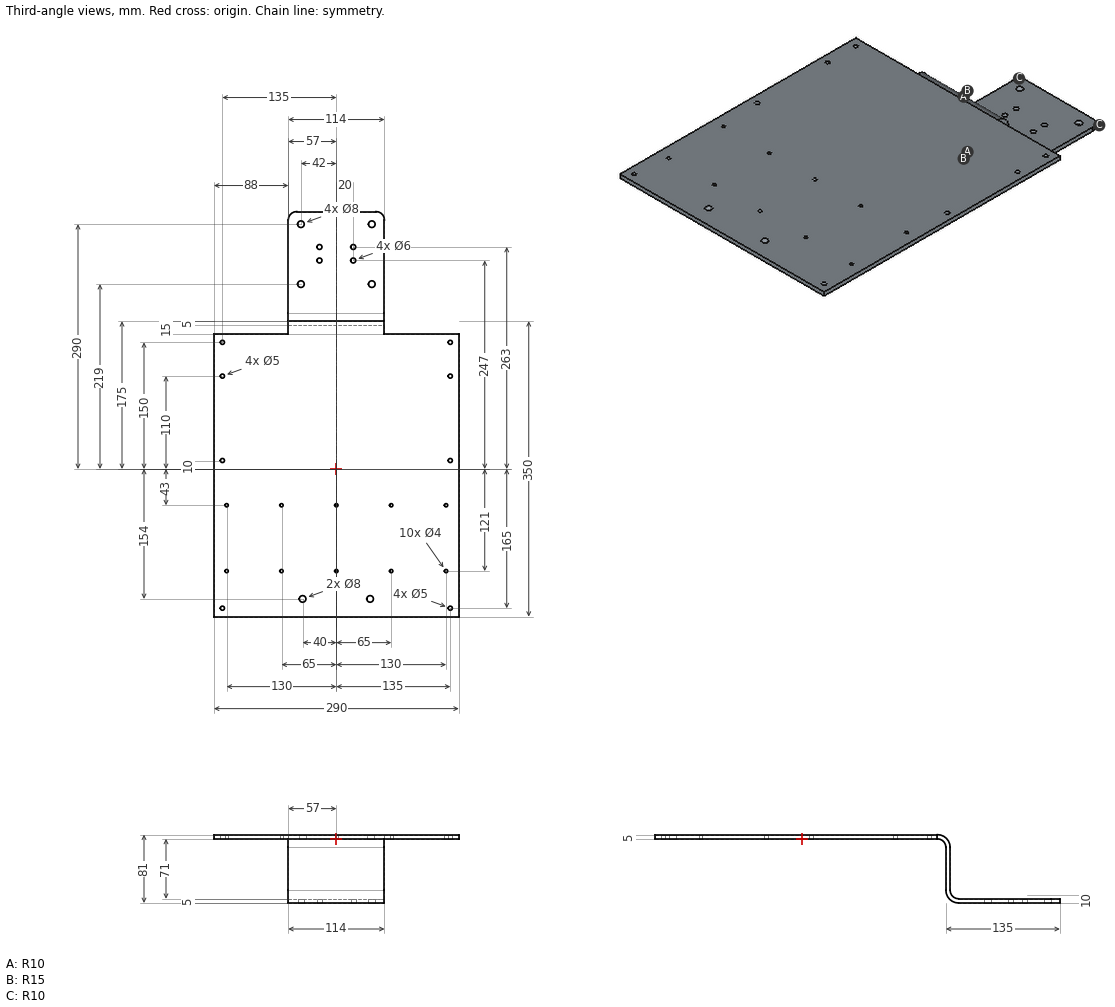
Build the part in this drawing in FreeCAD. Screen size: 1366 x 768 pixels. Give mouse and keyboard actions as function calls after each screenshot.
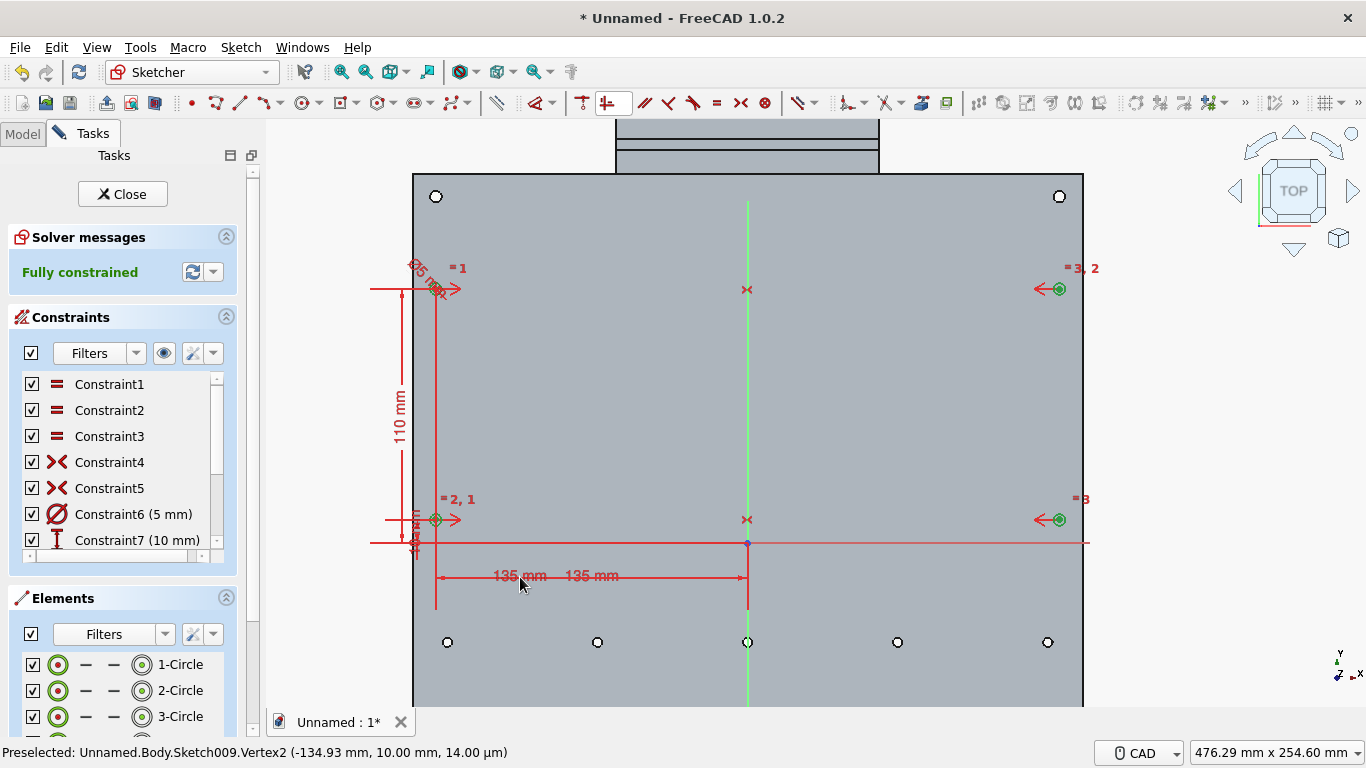
click(123, 194)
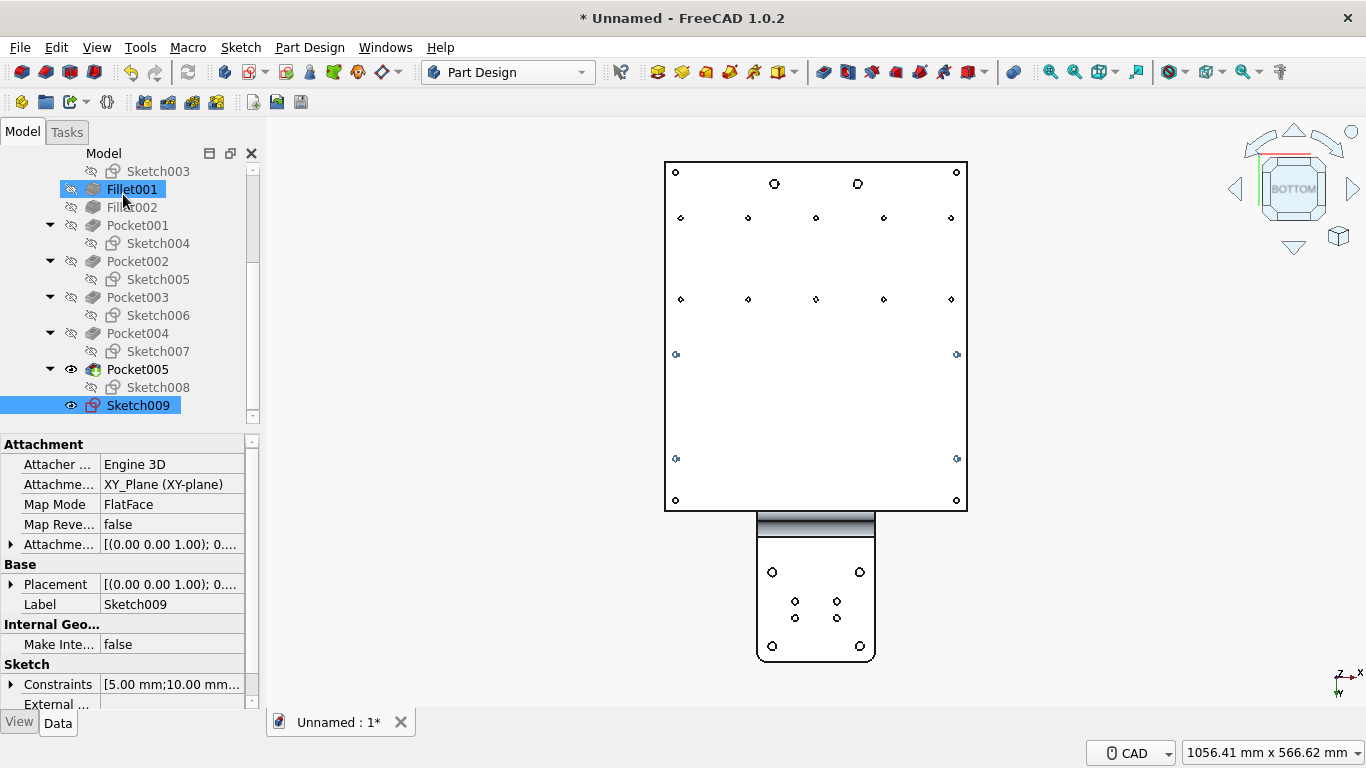
click(824, 72)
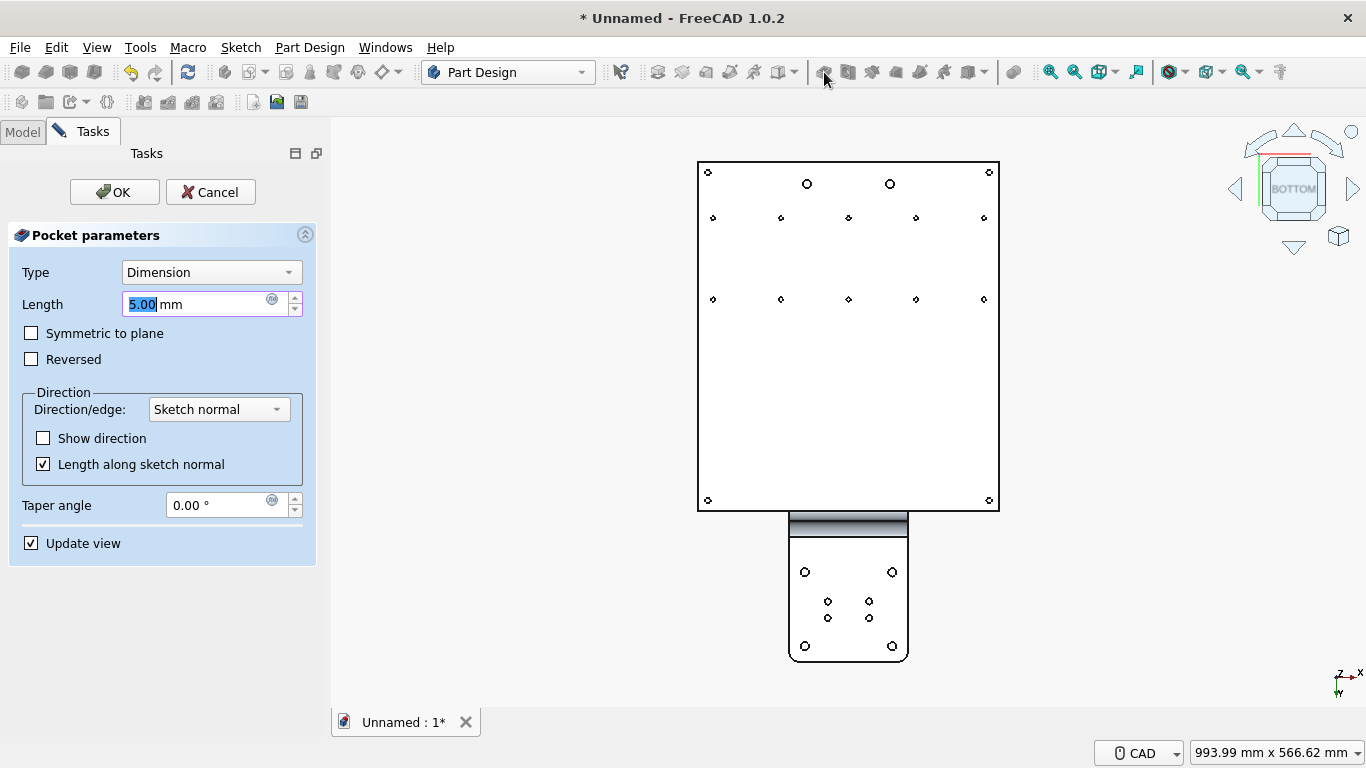
text(10)
key(Tab)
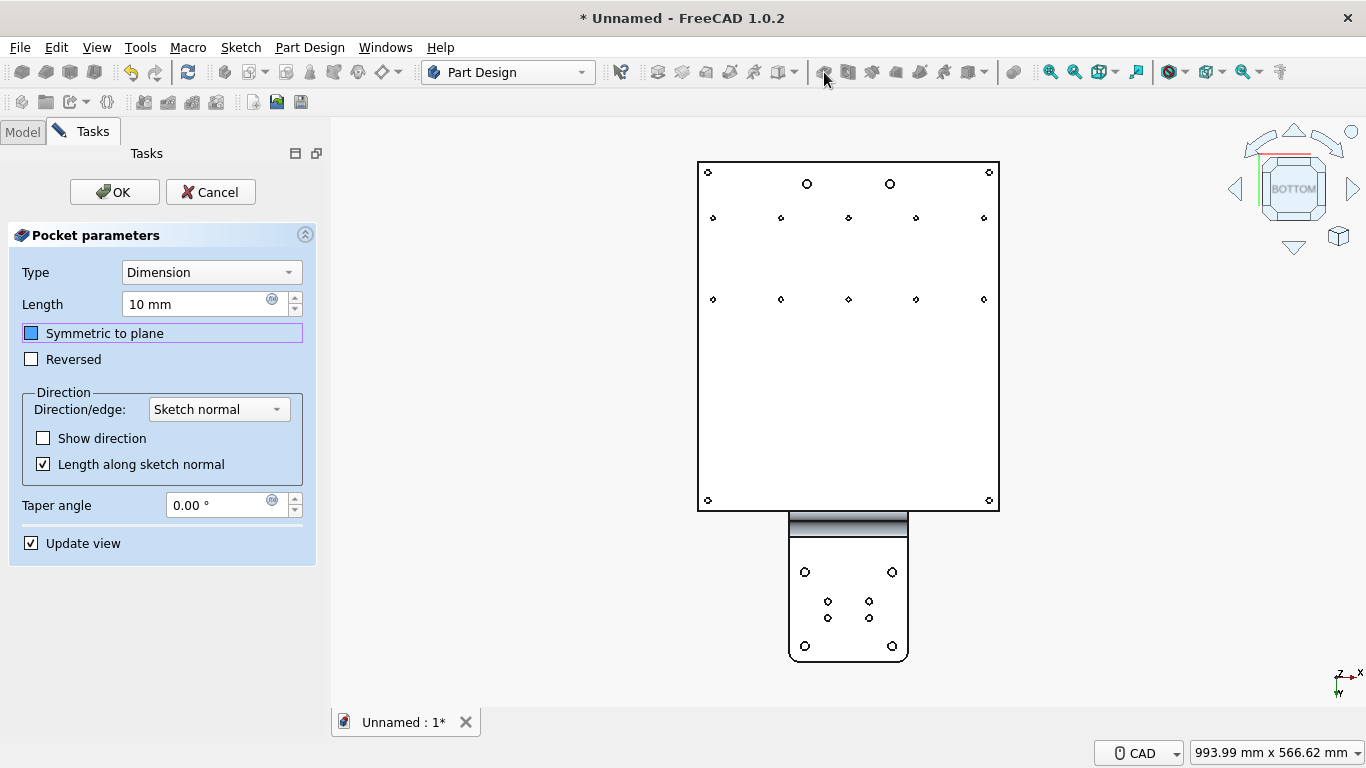
click(30, 359)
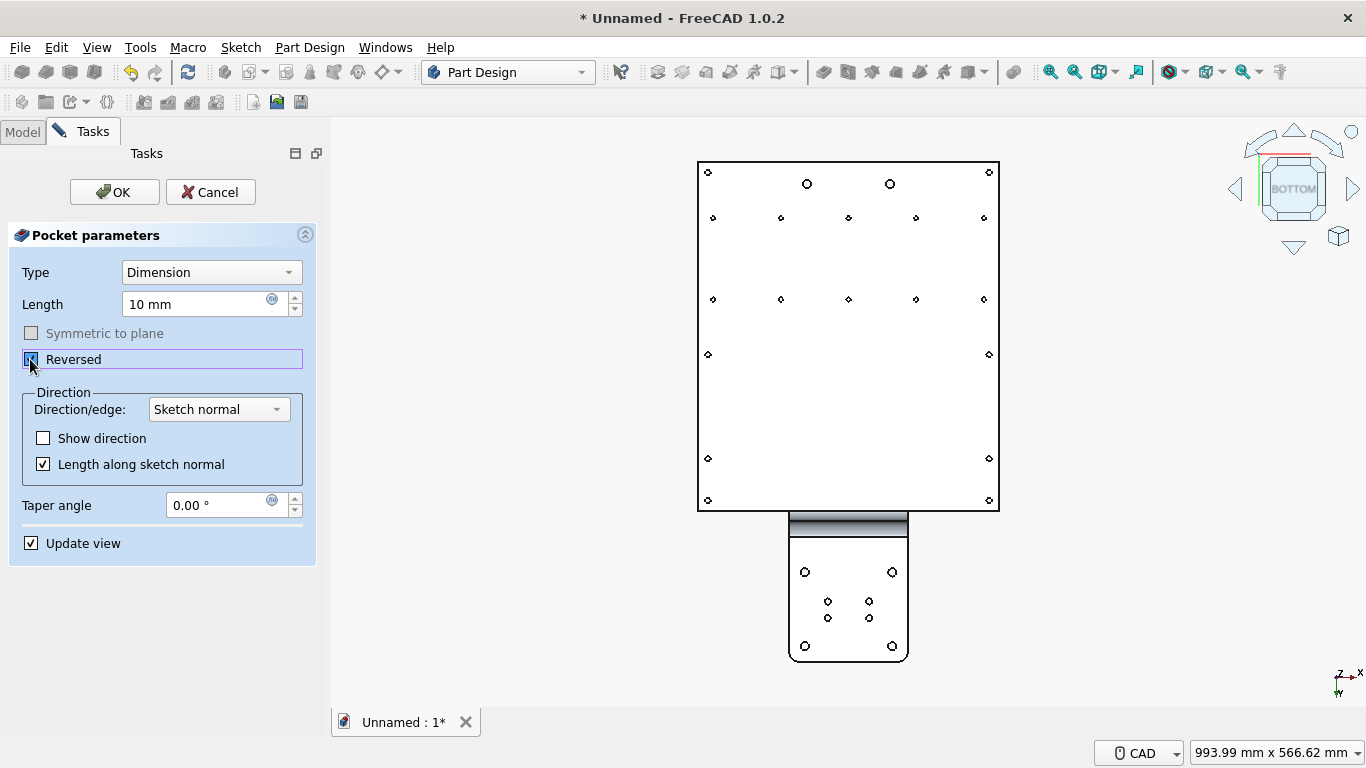
click(115, 192)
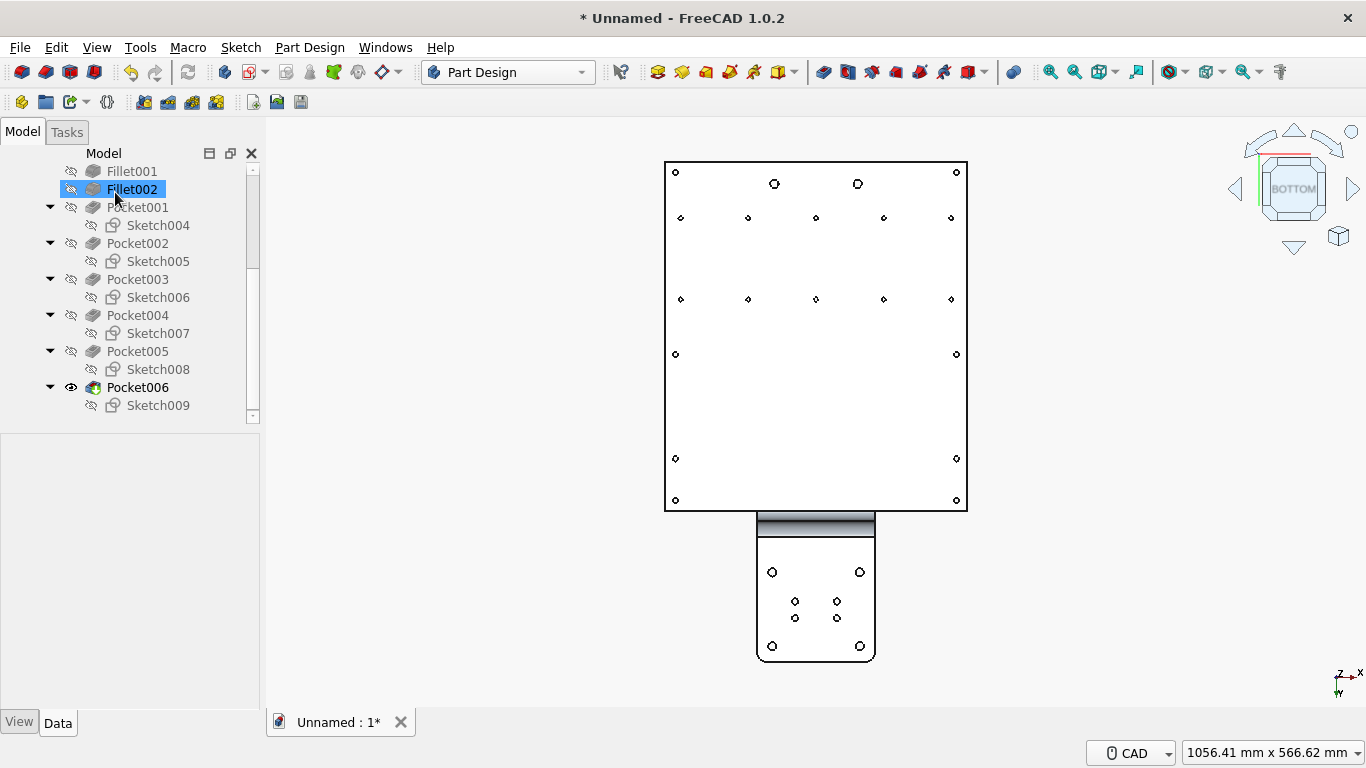
key(0)